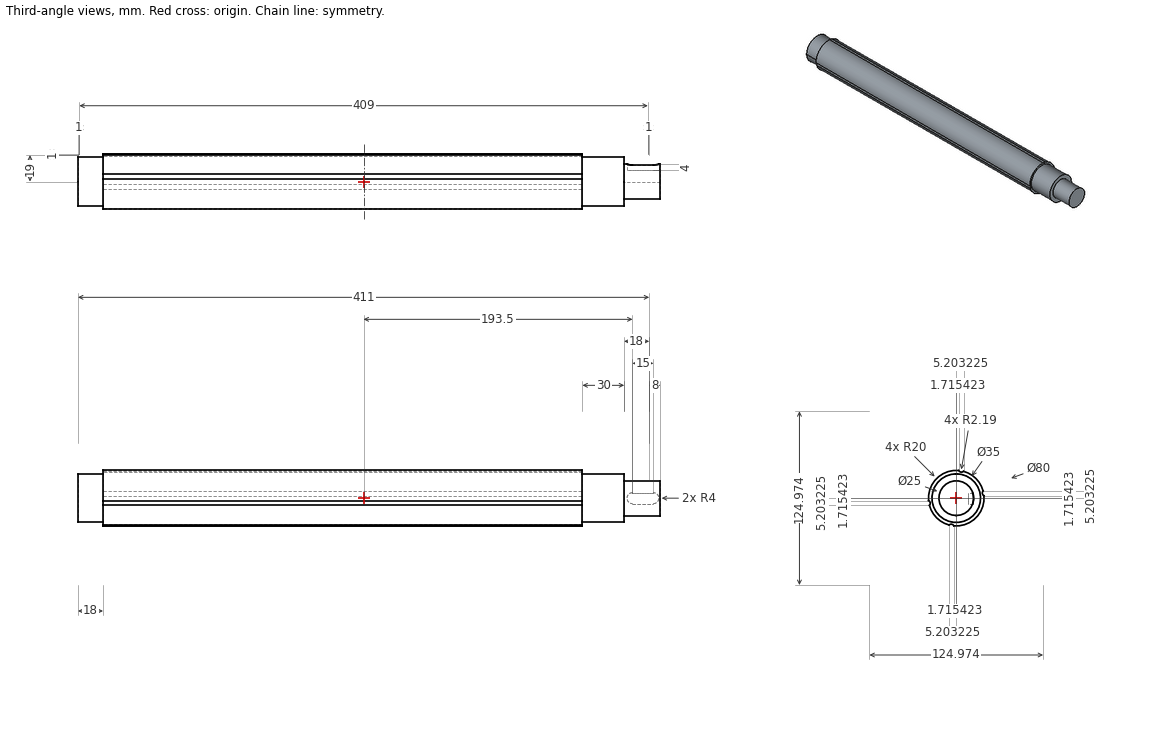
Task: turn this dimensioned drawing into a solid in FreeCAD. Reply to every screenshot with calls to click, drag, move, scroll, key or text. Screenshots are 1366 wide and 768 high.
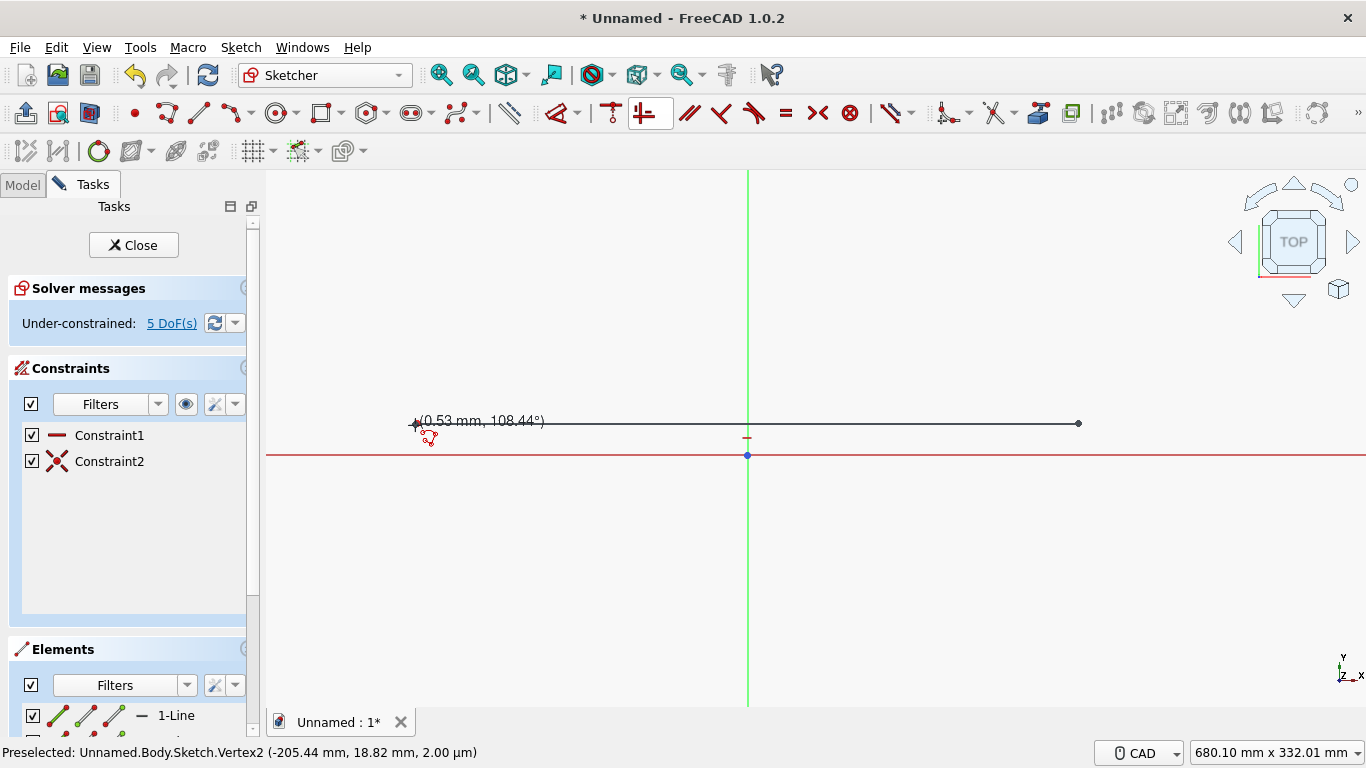
click(415, 455)
click(1080, 446)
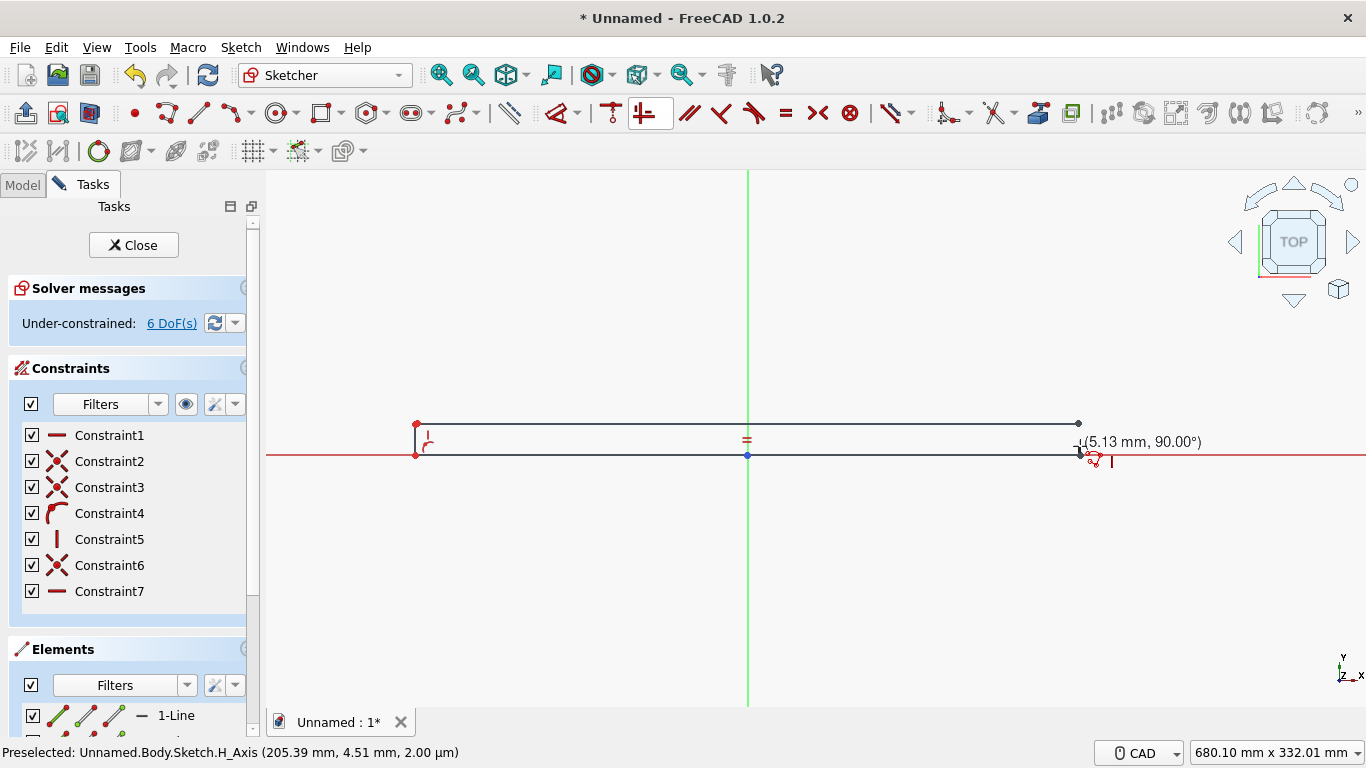
scroll(1080, 425, up, 10)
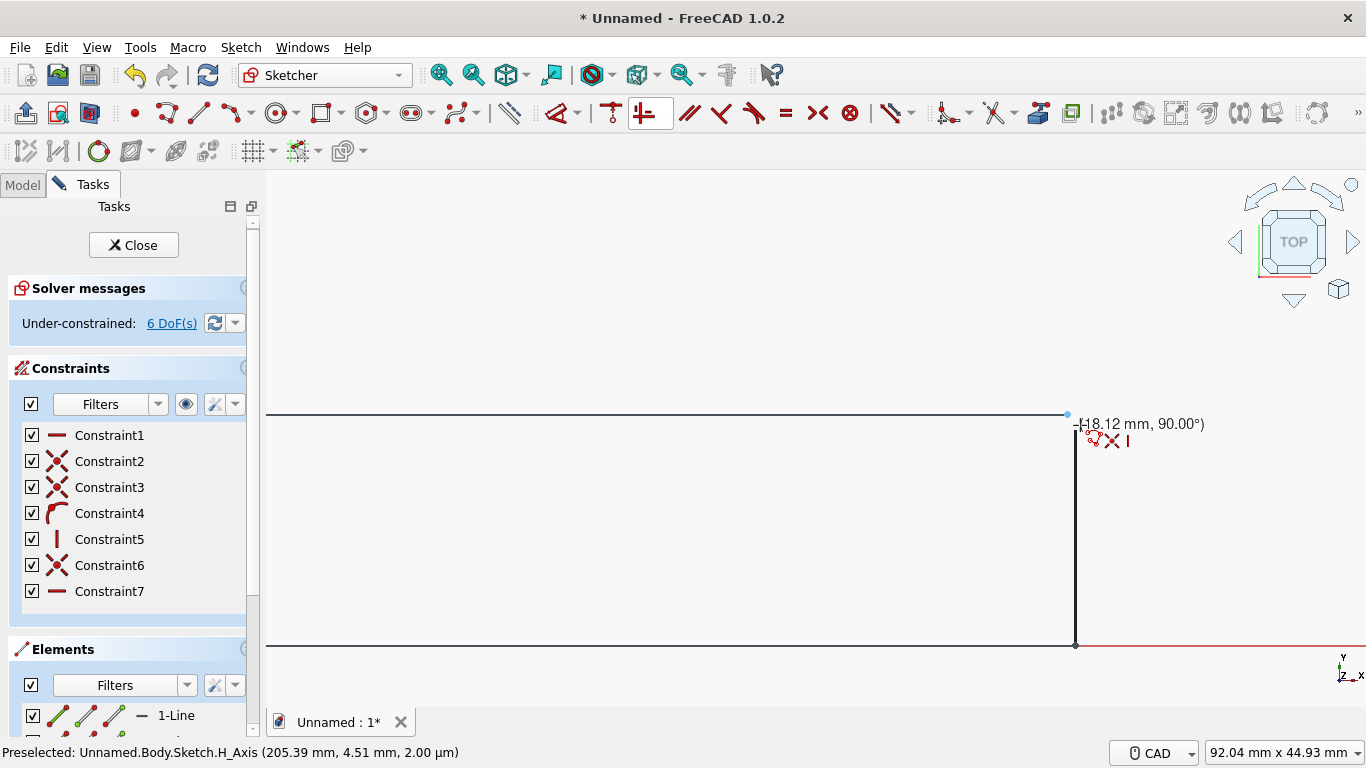
click(1075, 419)
click(1068, 415)
key(Escape)
key(Escape)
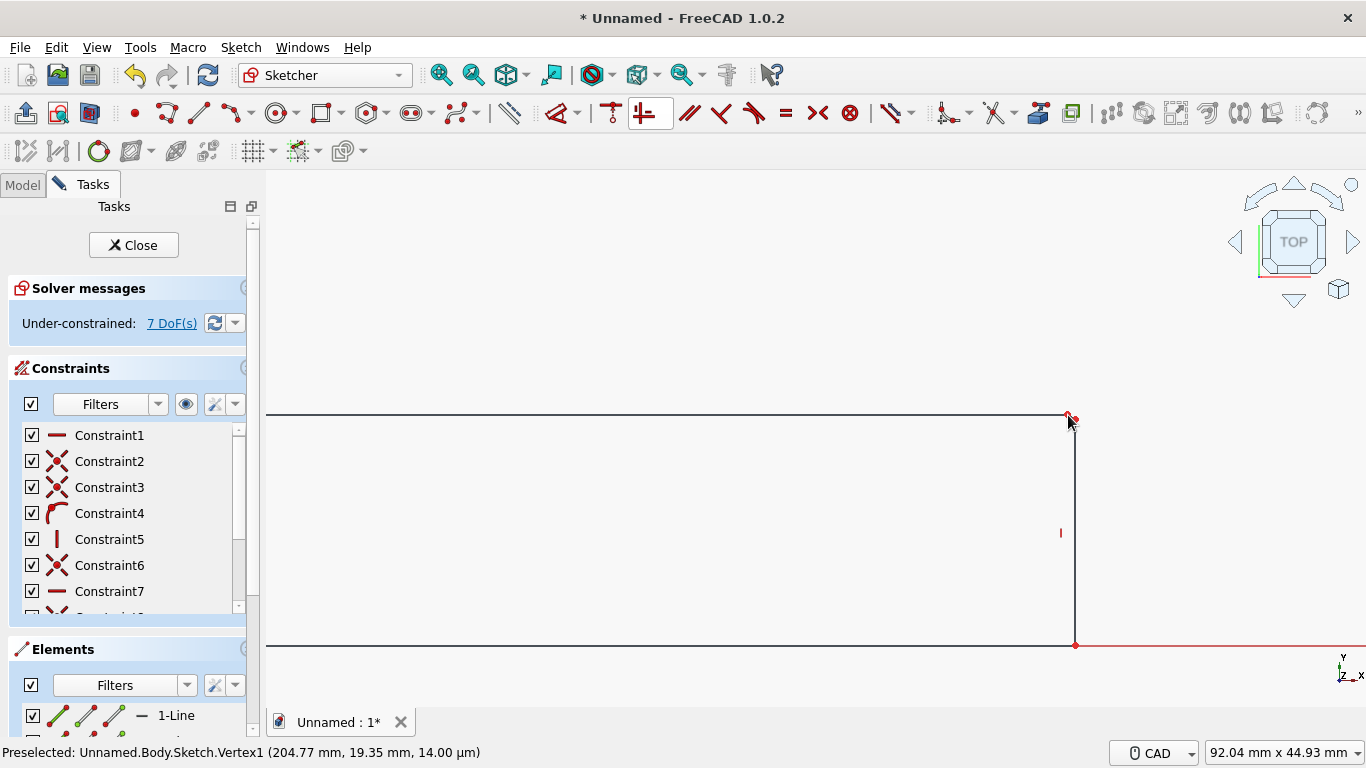
scroll(1080, 425, down, 10)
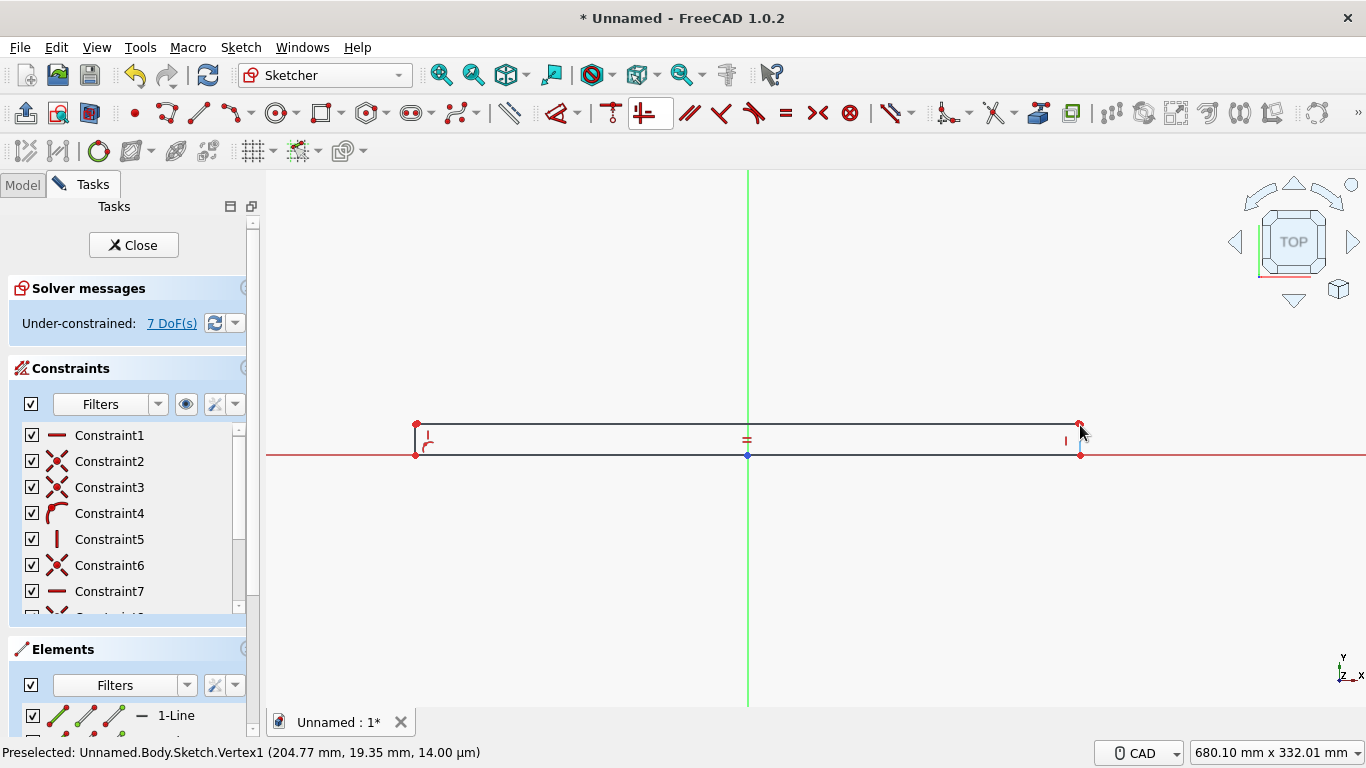
scroll(415, 425, up, 10)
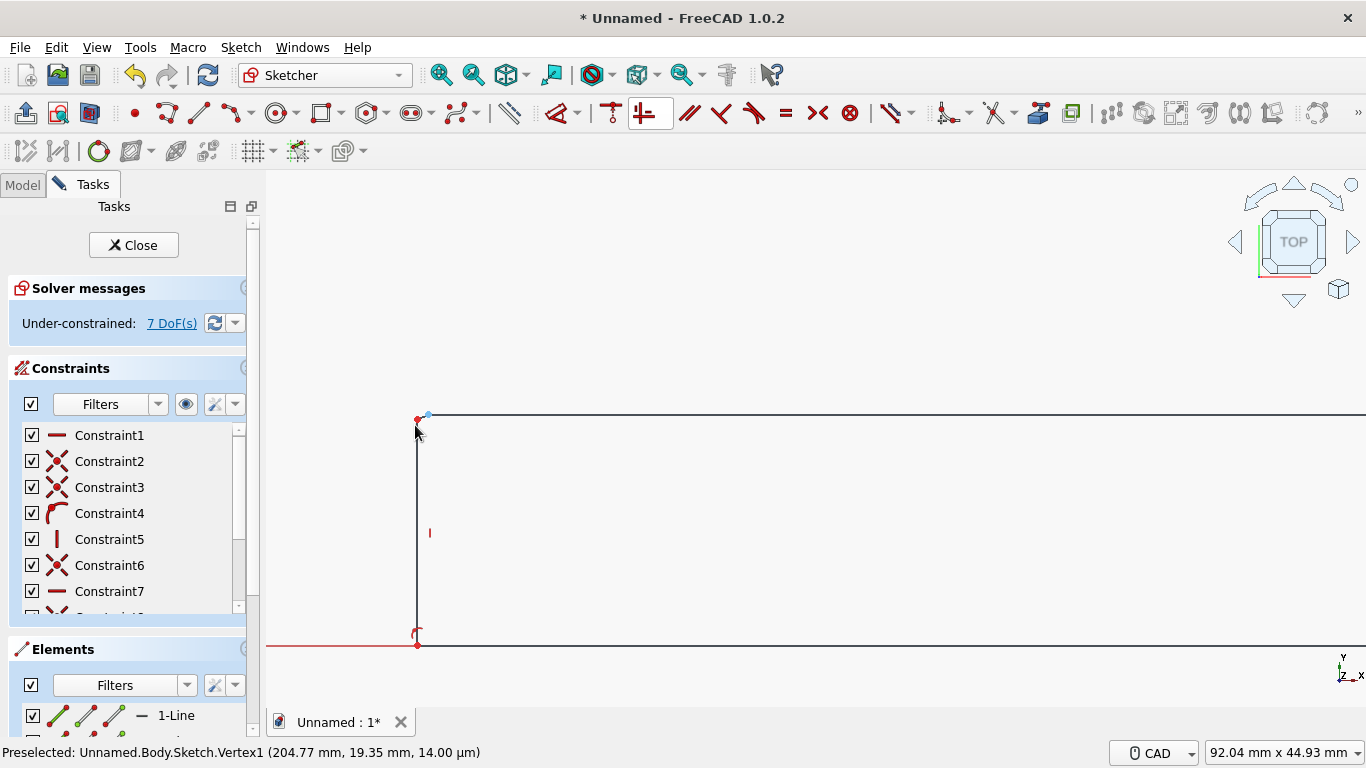
click(417, 420)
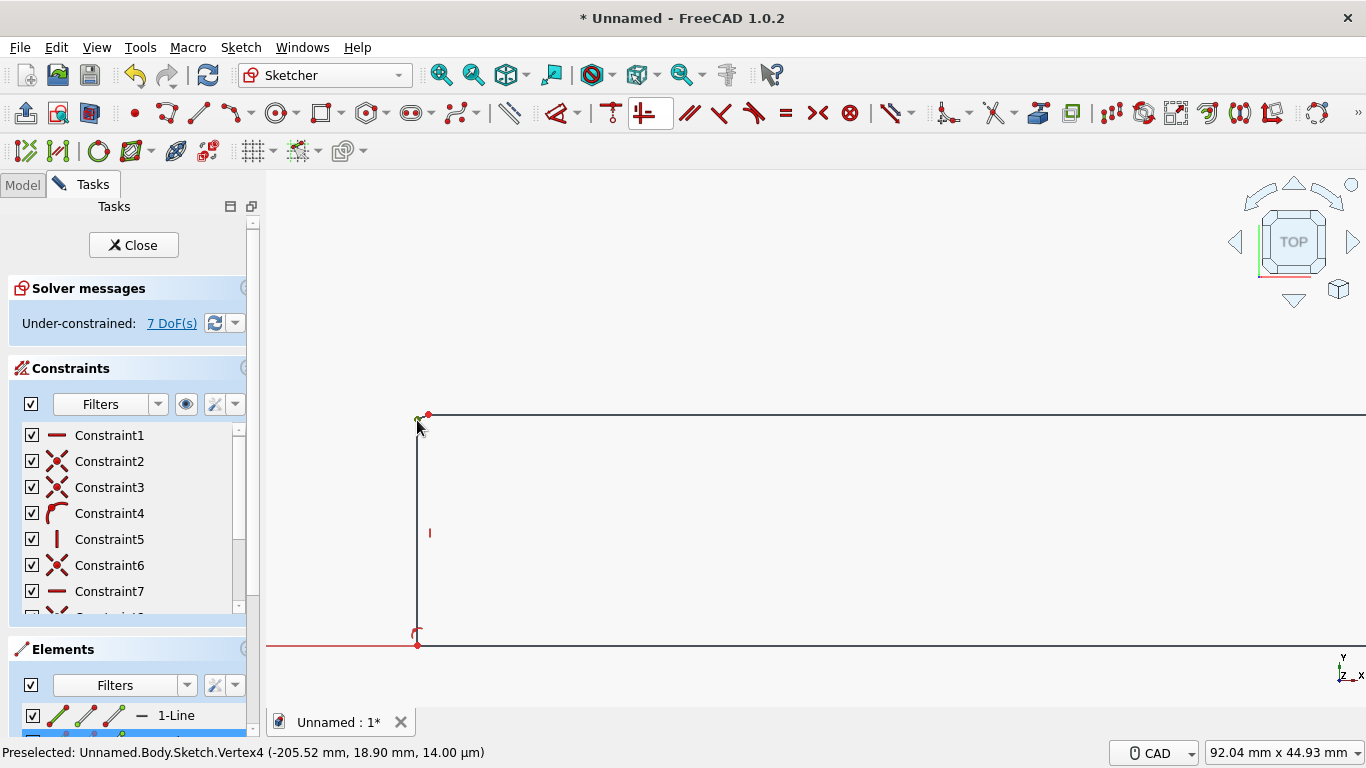
scroll(415, 425, down, 10)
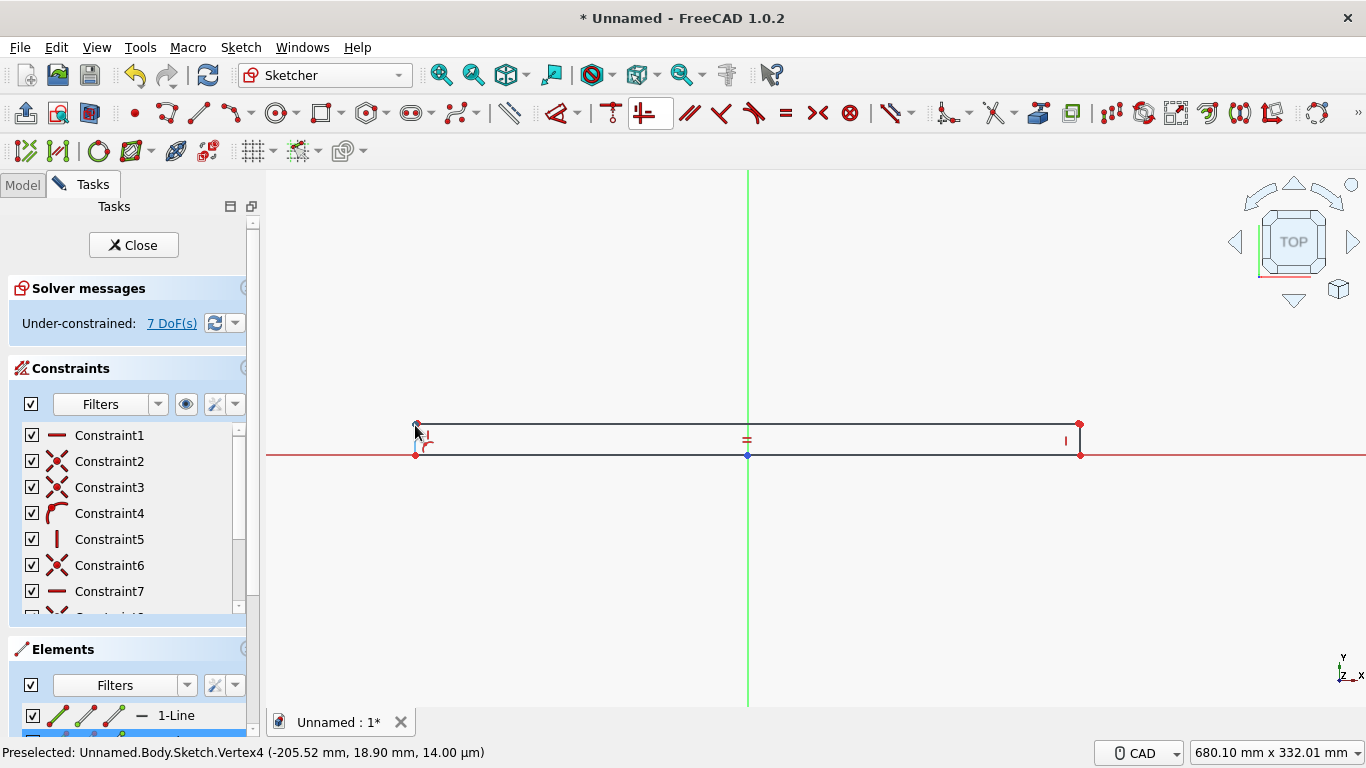
scroll(1080, 425, up, 12)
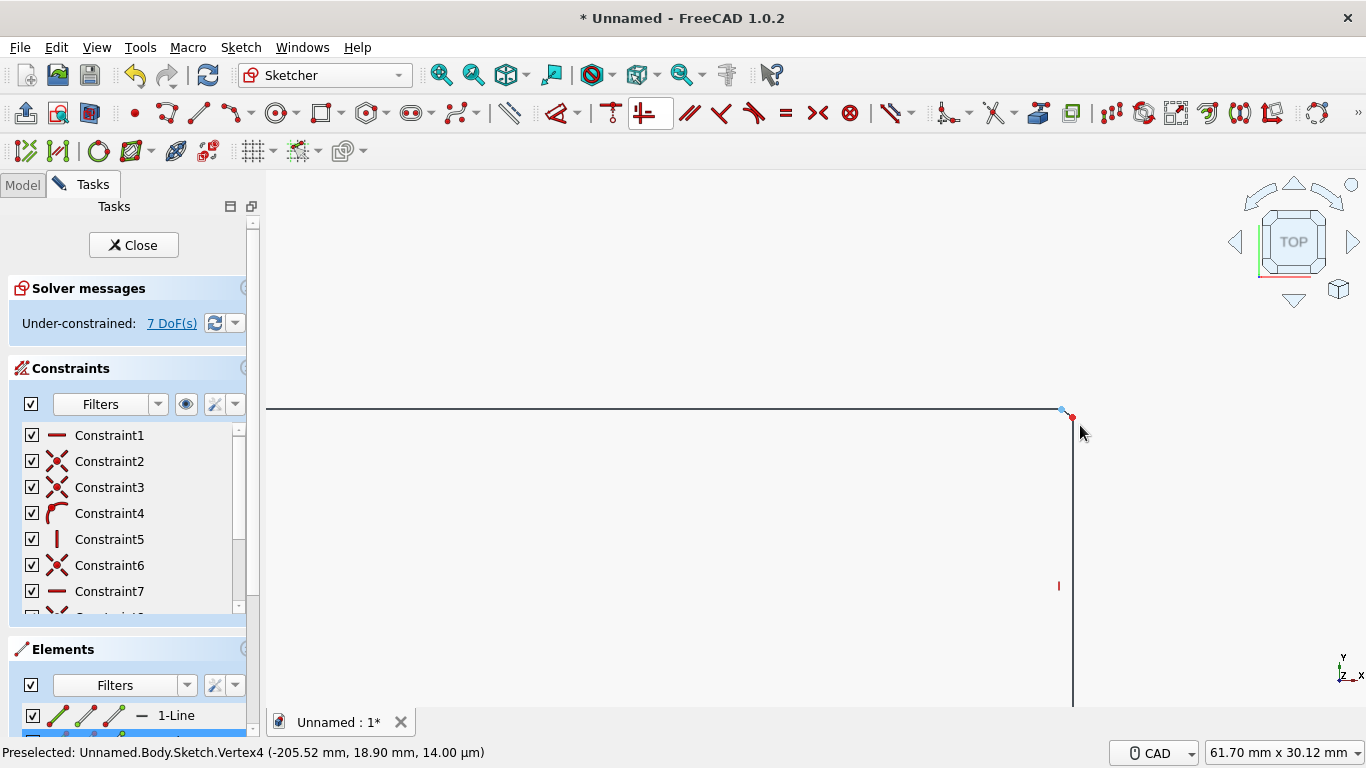
click(1073, 417)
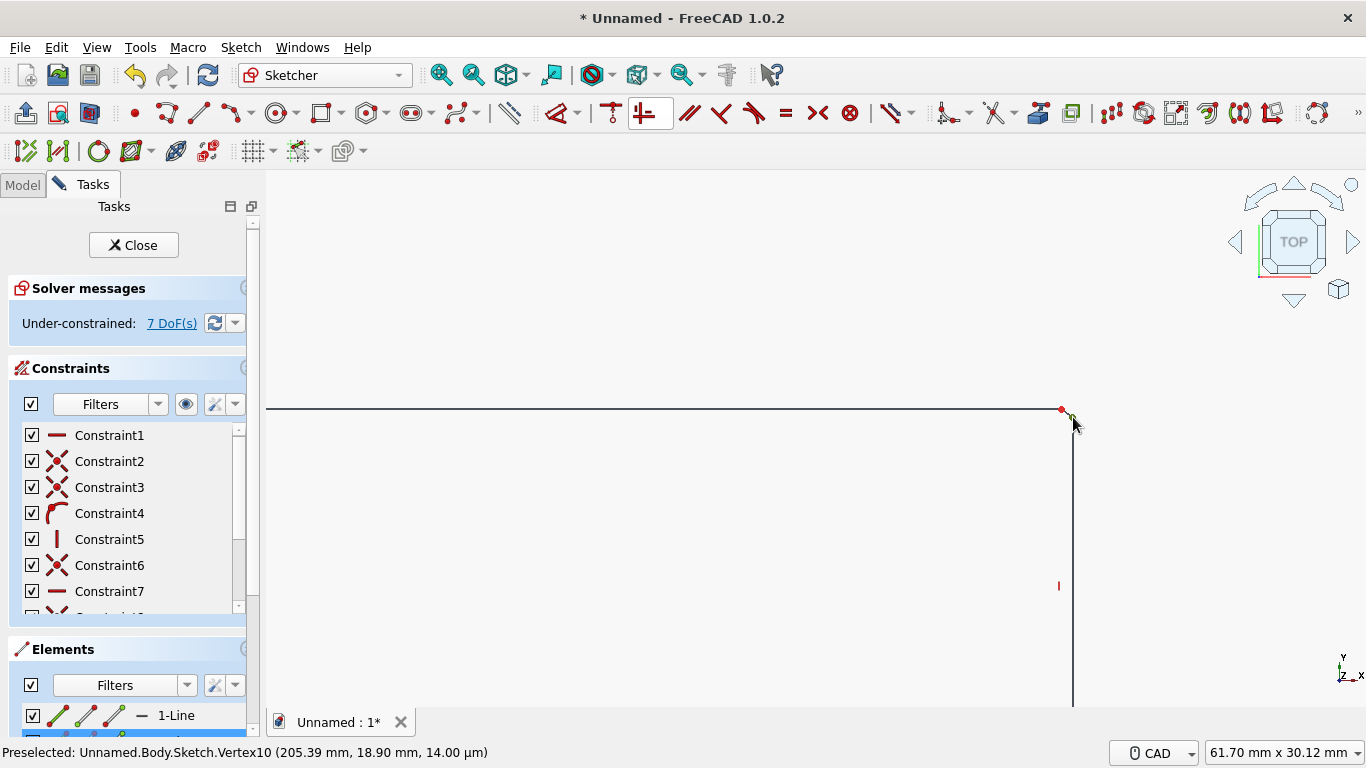
scroll(1080, 425, down, 12)